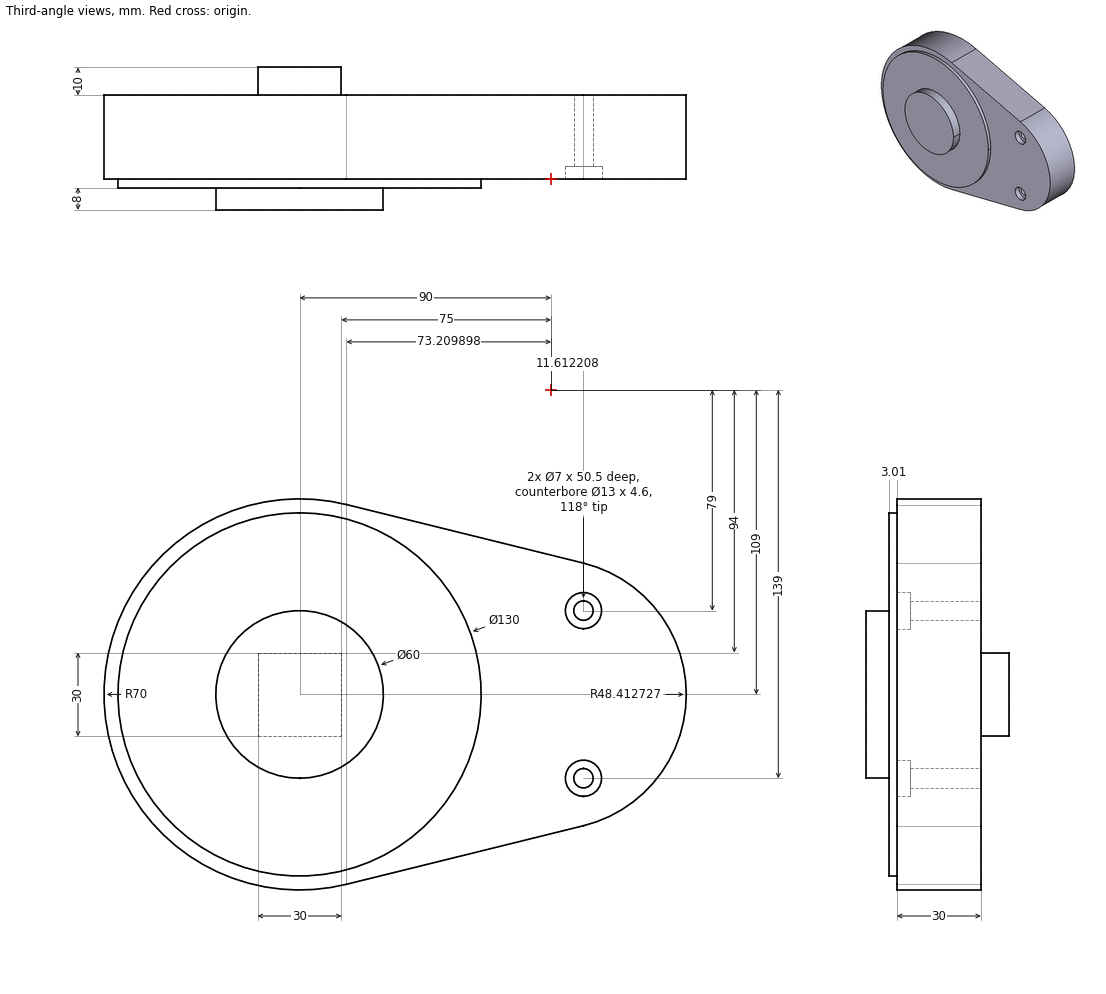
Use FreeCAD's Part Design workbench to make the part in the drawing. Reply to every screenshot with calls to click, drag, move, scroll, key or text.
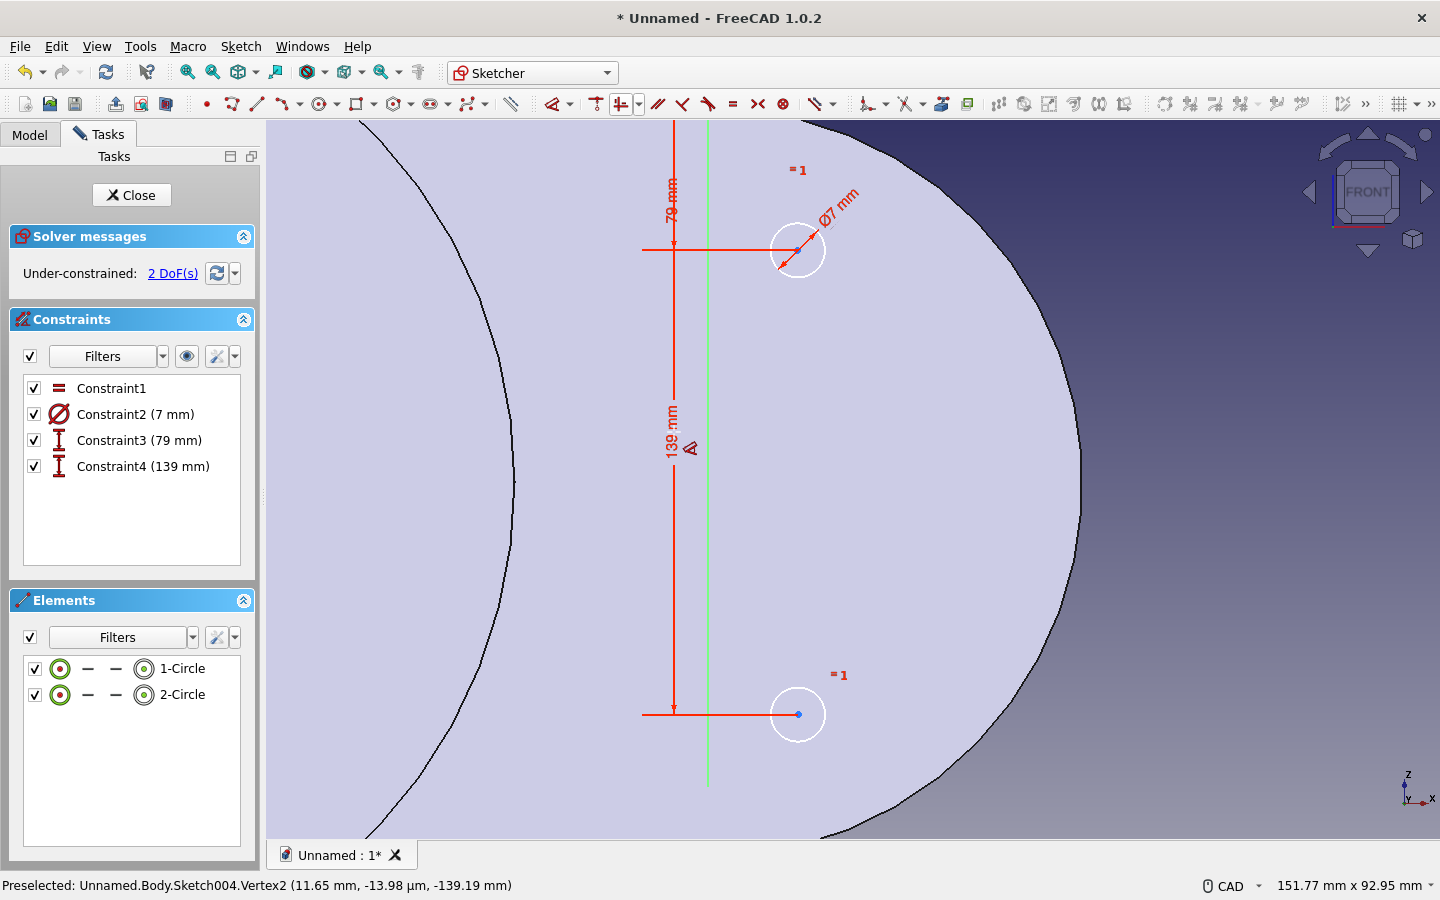
click(798, 250)
click(753, 284)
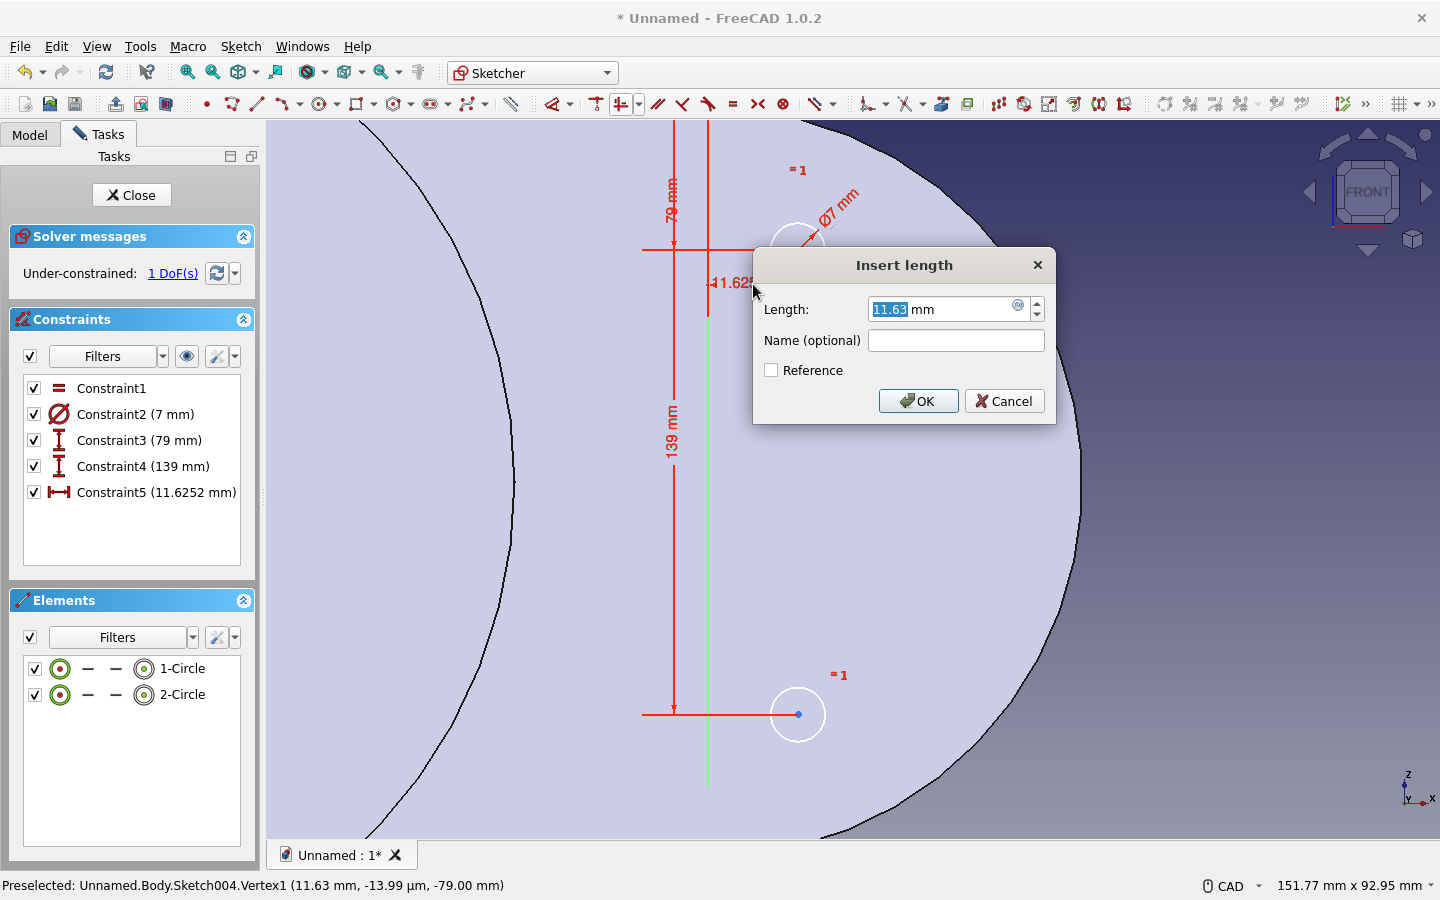
text(11.612208)
key(Return)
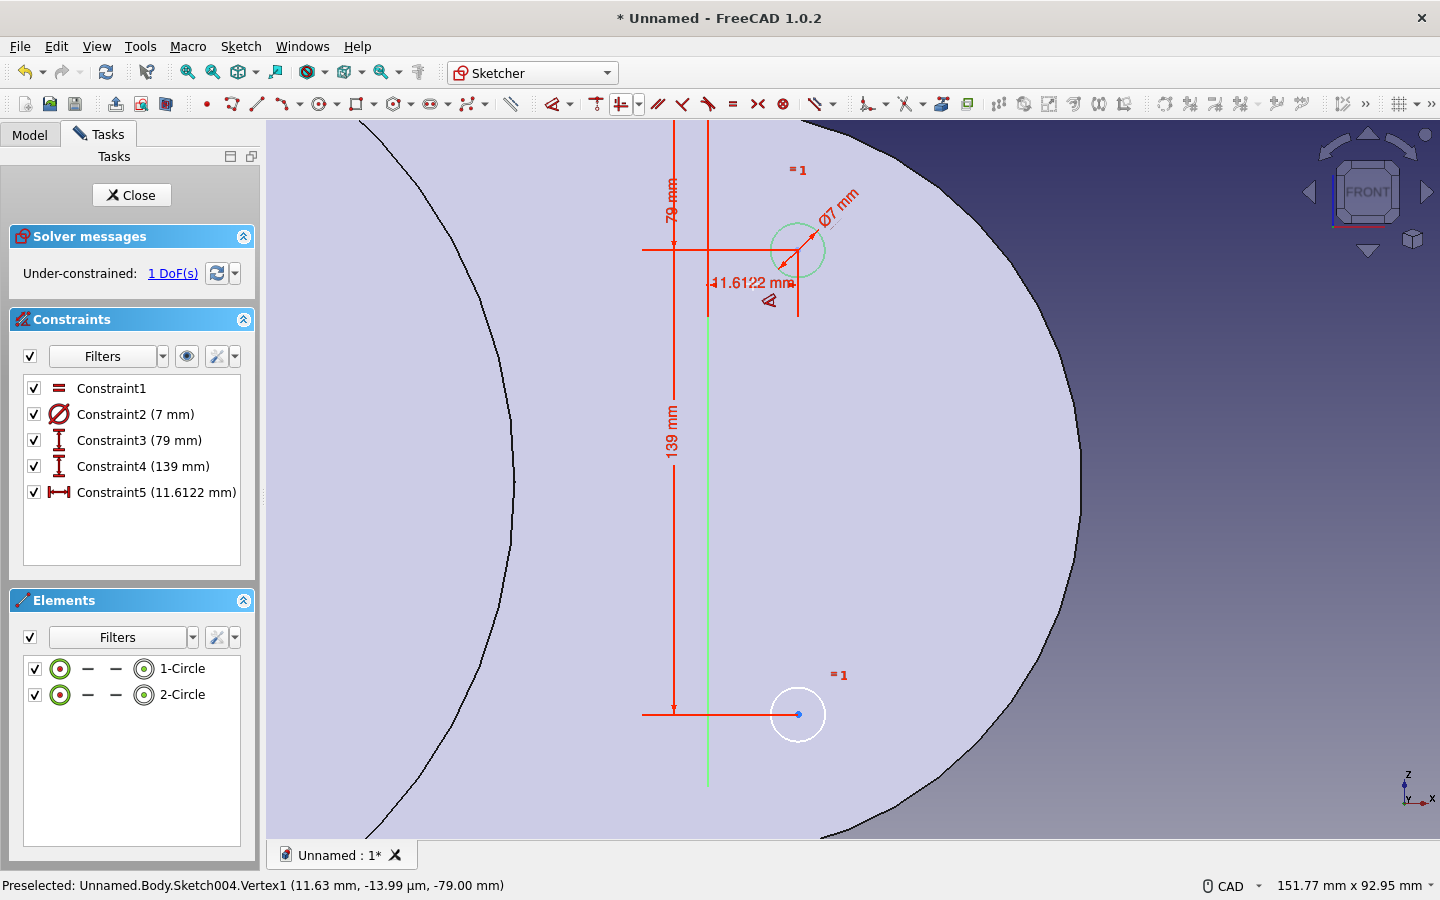
click(798, 715)
click(753, 749)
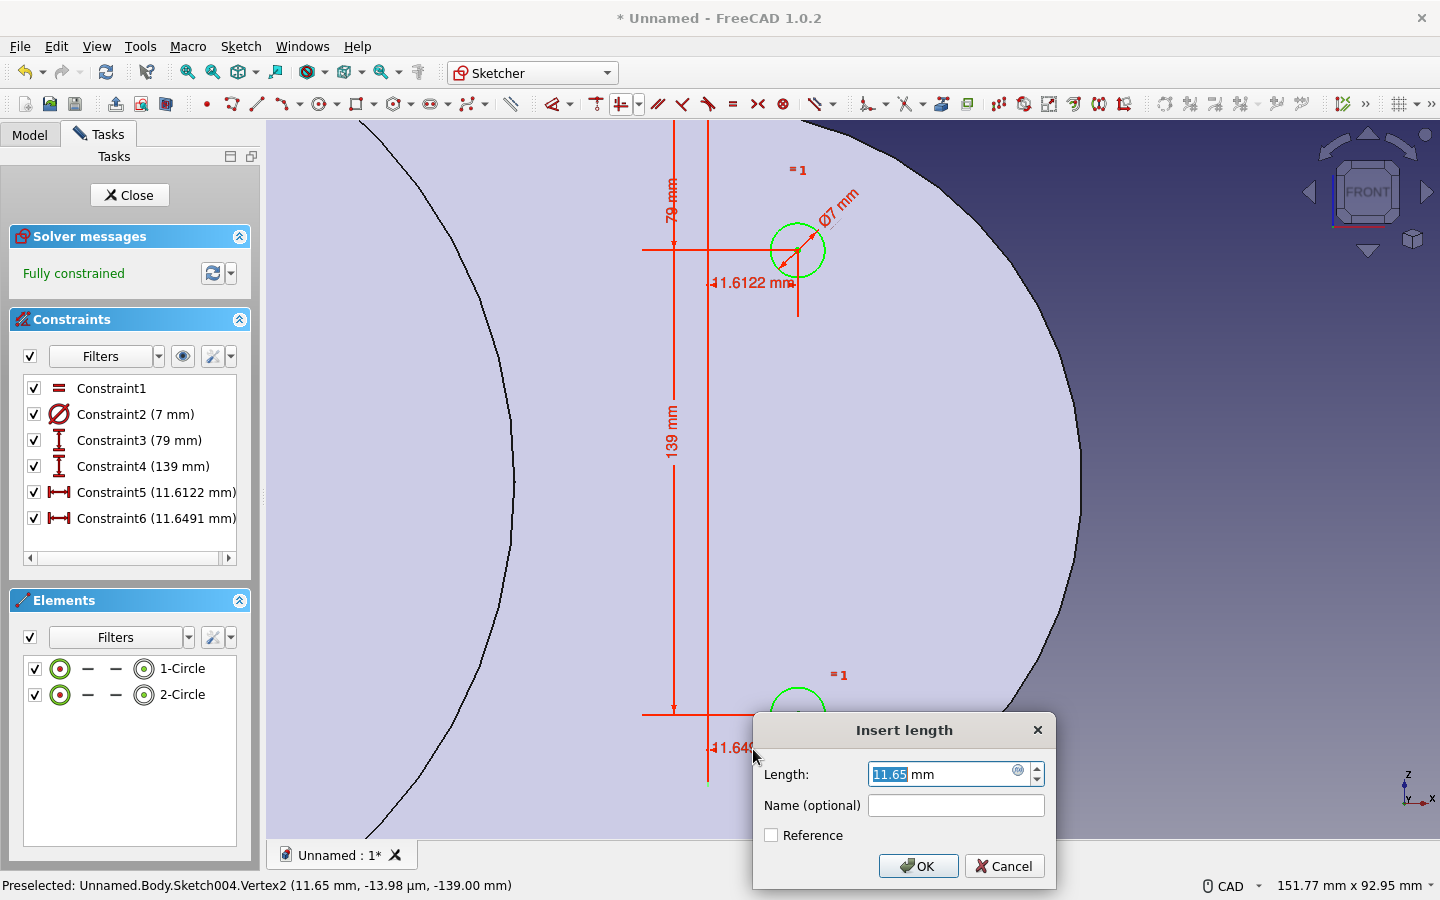
text(11.612208)
key(Return)
key(Escape)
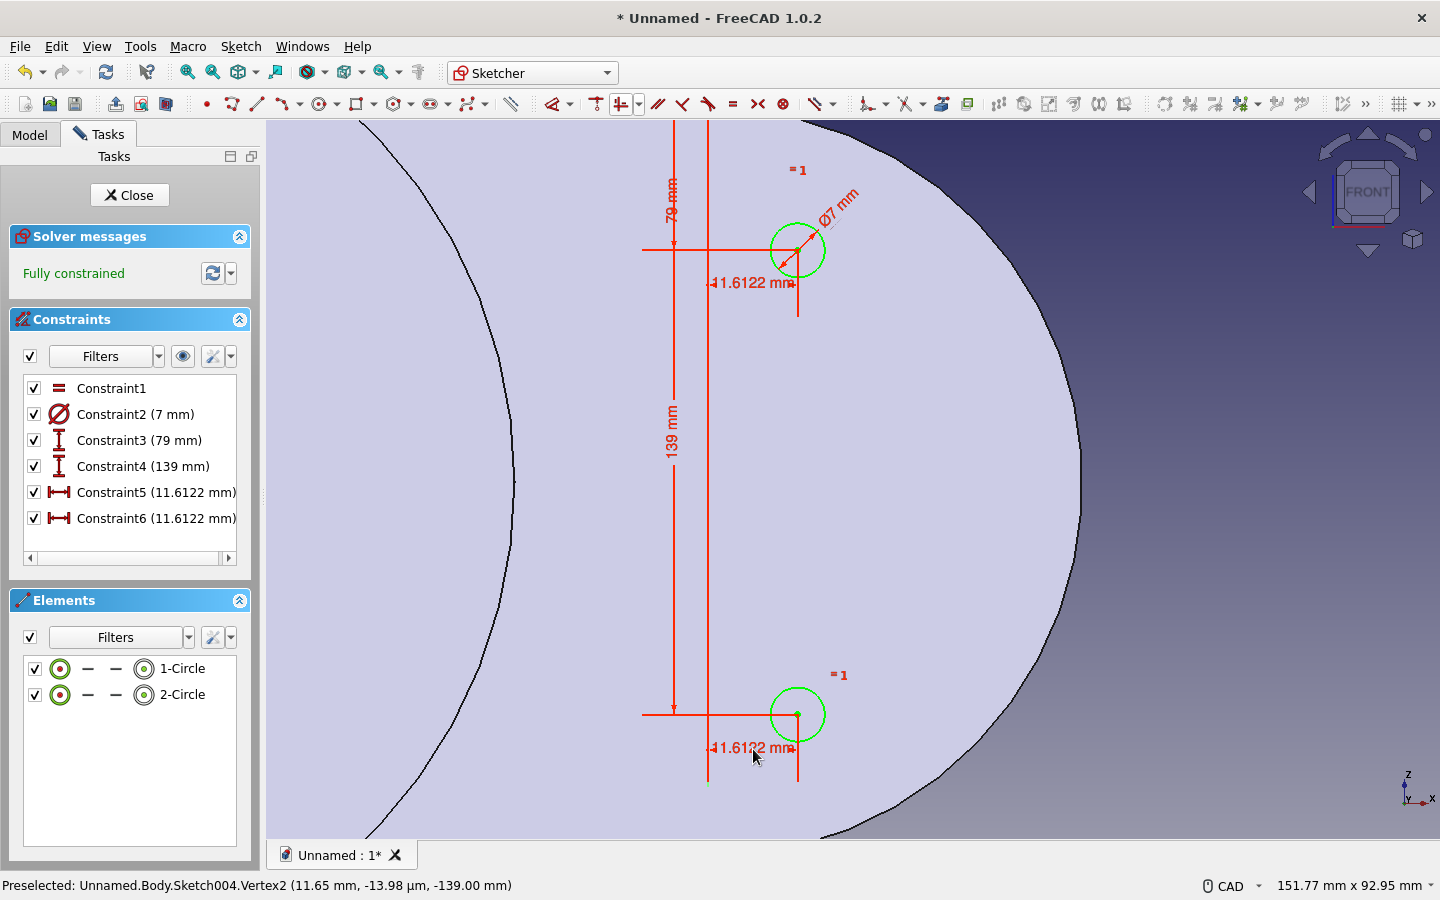
click(130, 195)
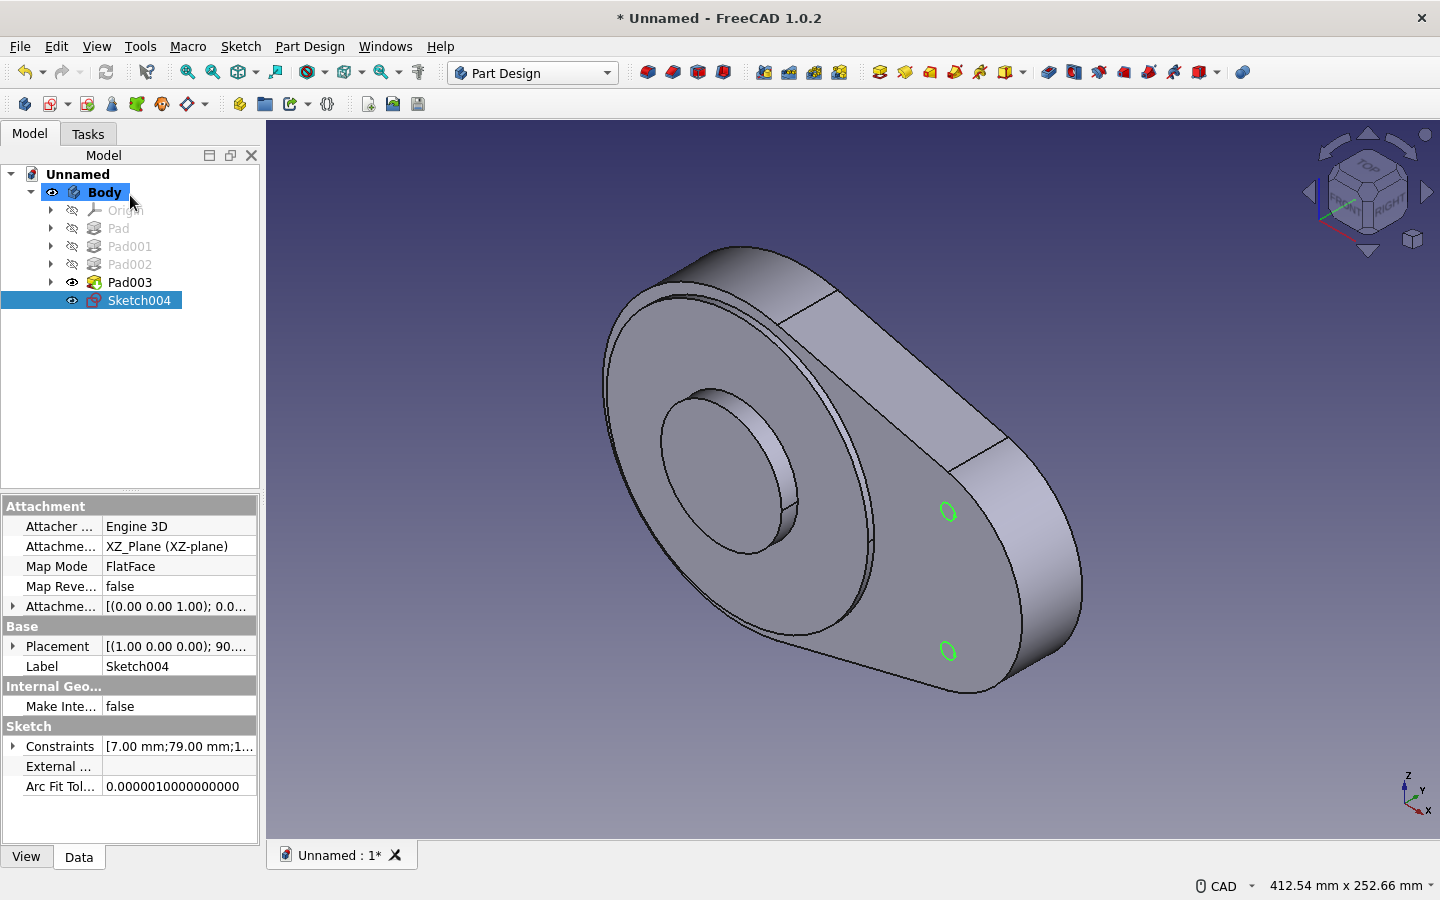
click(1074, 72)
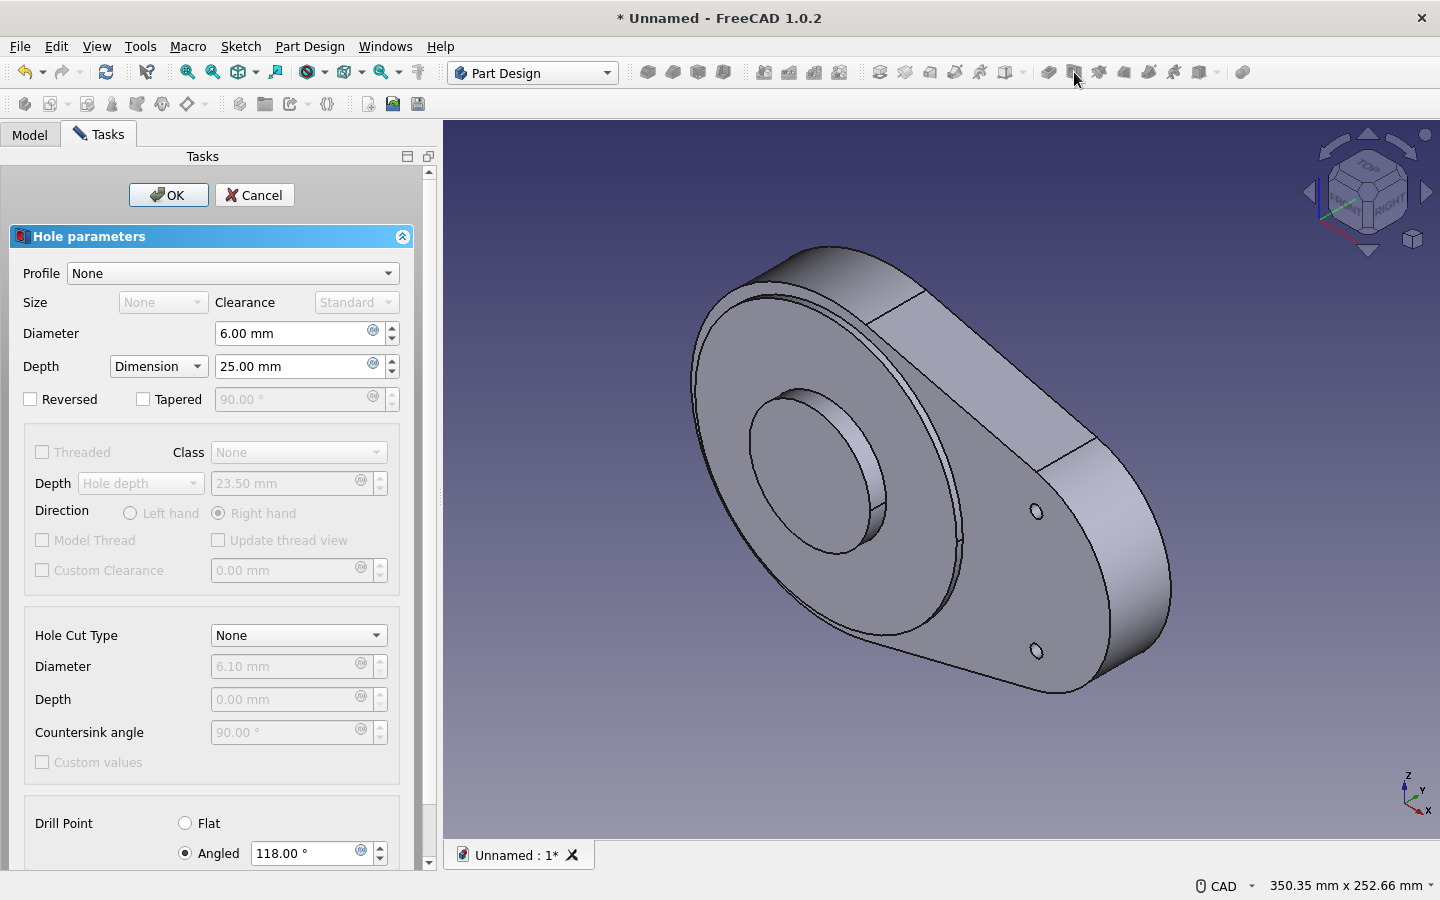
triple_click(300, 334)